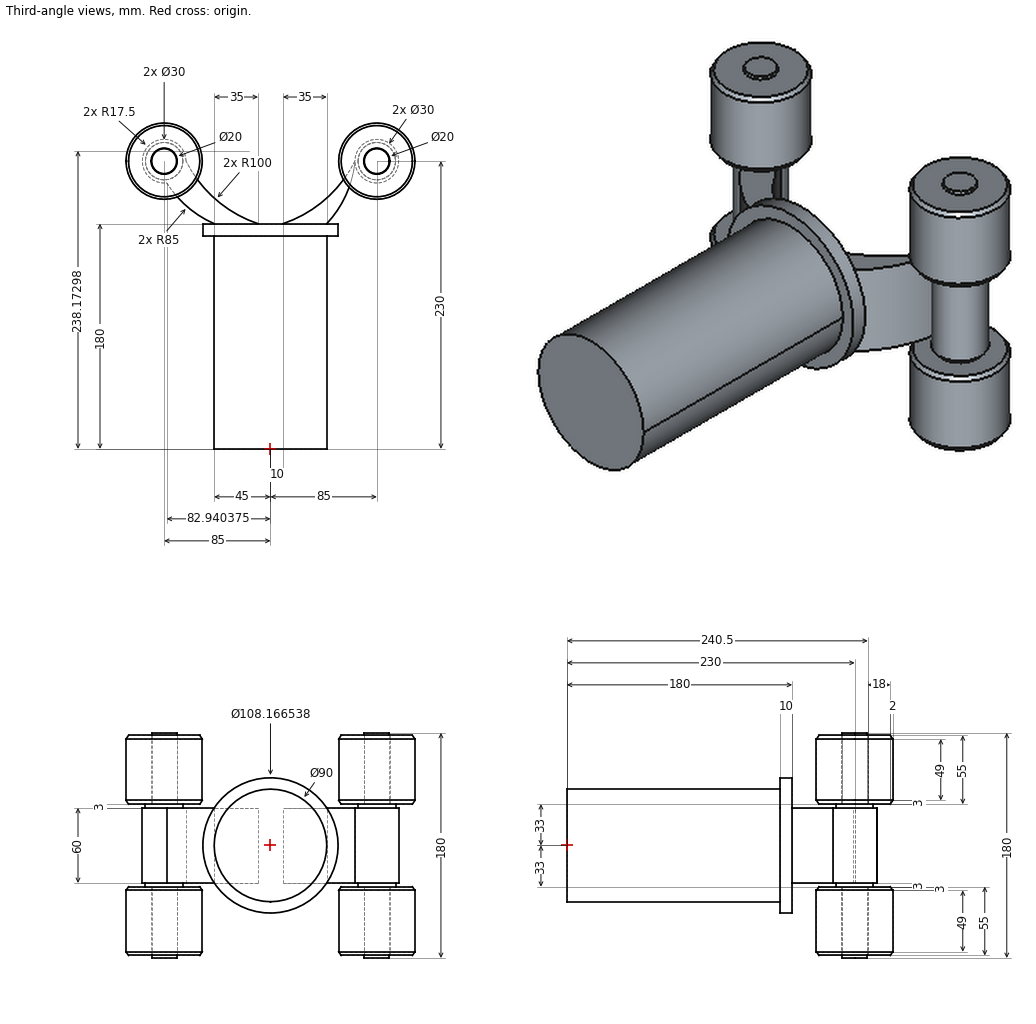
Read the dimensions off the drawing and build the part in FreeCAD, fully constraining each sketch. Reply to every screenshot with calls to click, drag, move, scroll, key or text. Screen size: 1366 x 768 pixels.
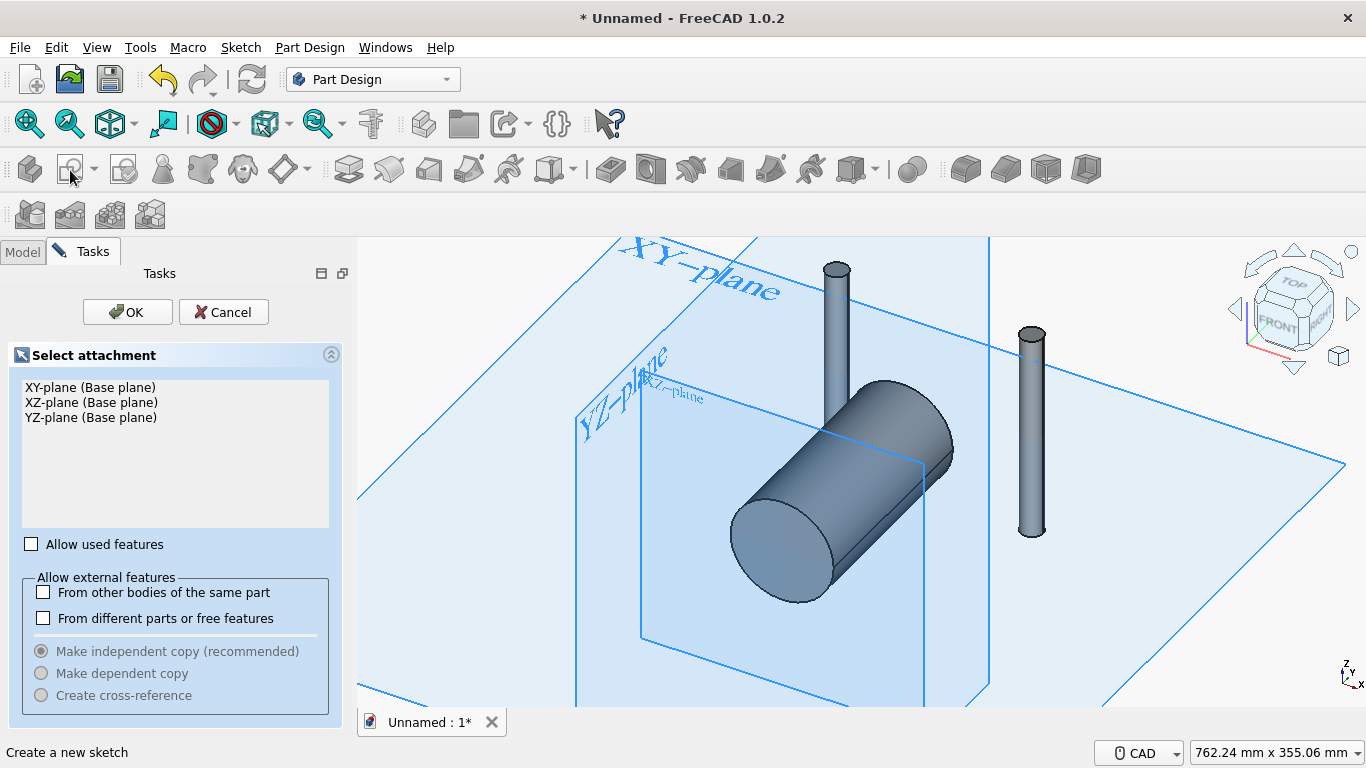
click(82, 388)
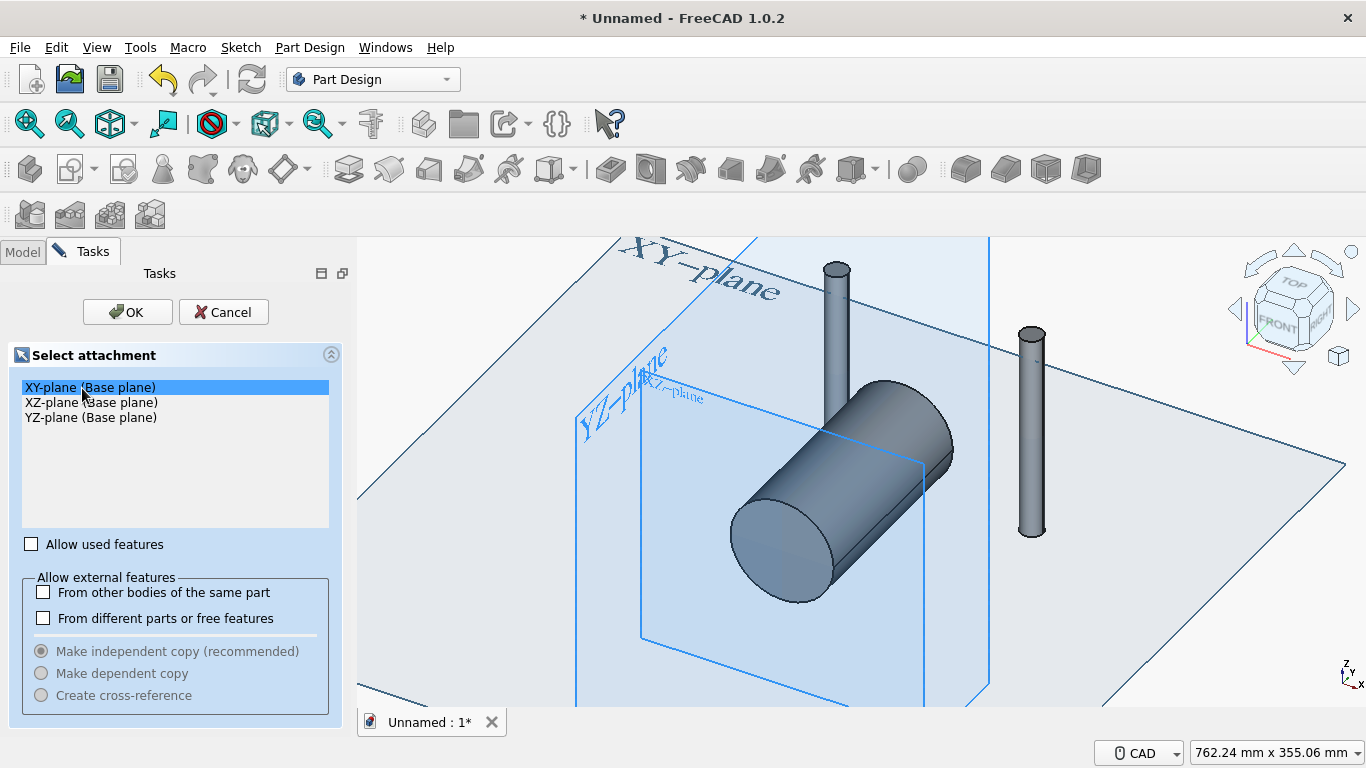
click(128, 312)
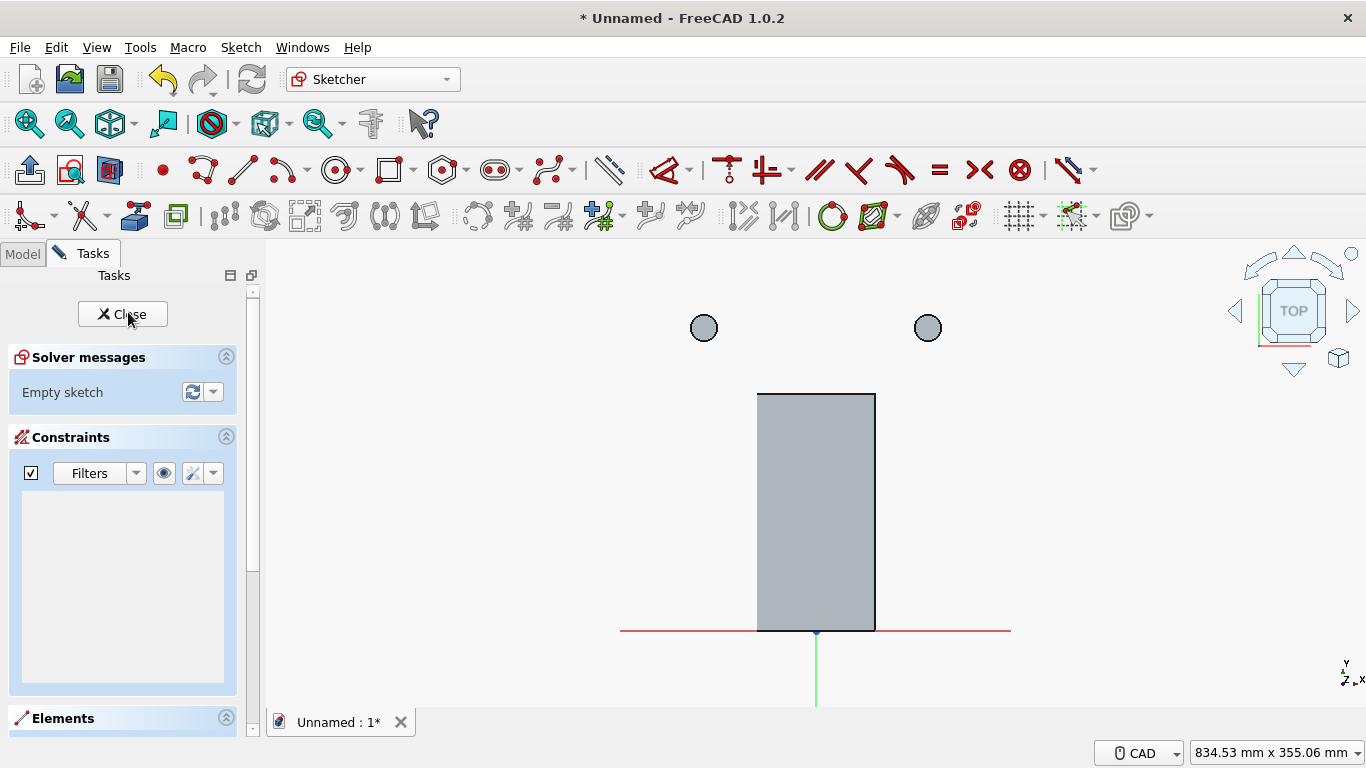
click(110, 170)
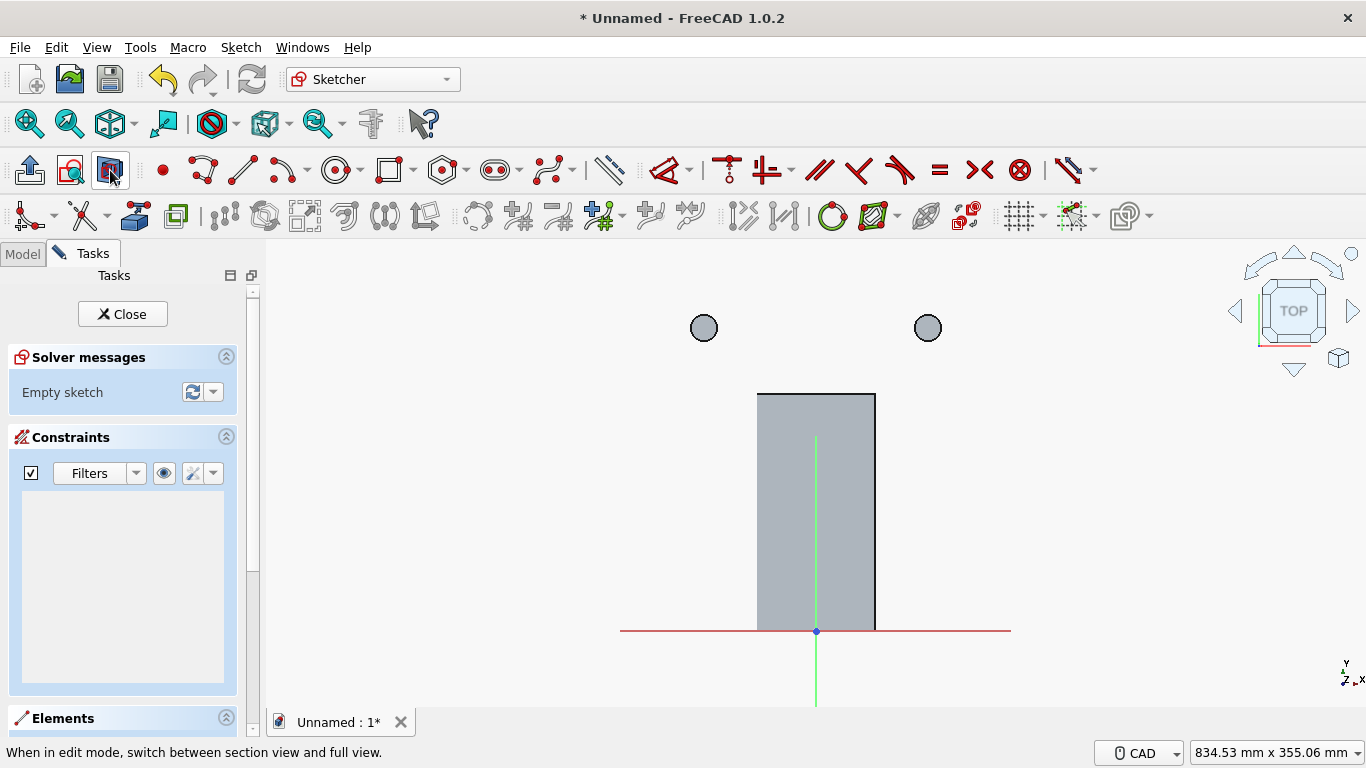
click(244, 170)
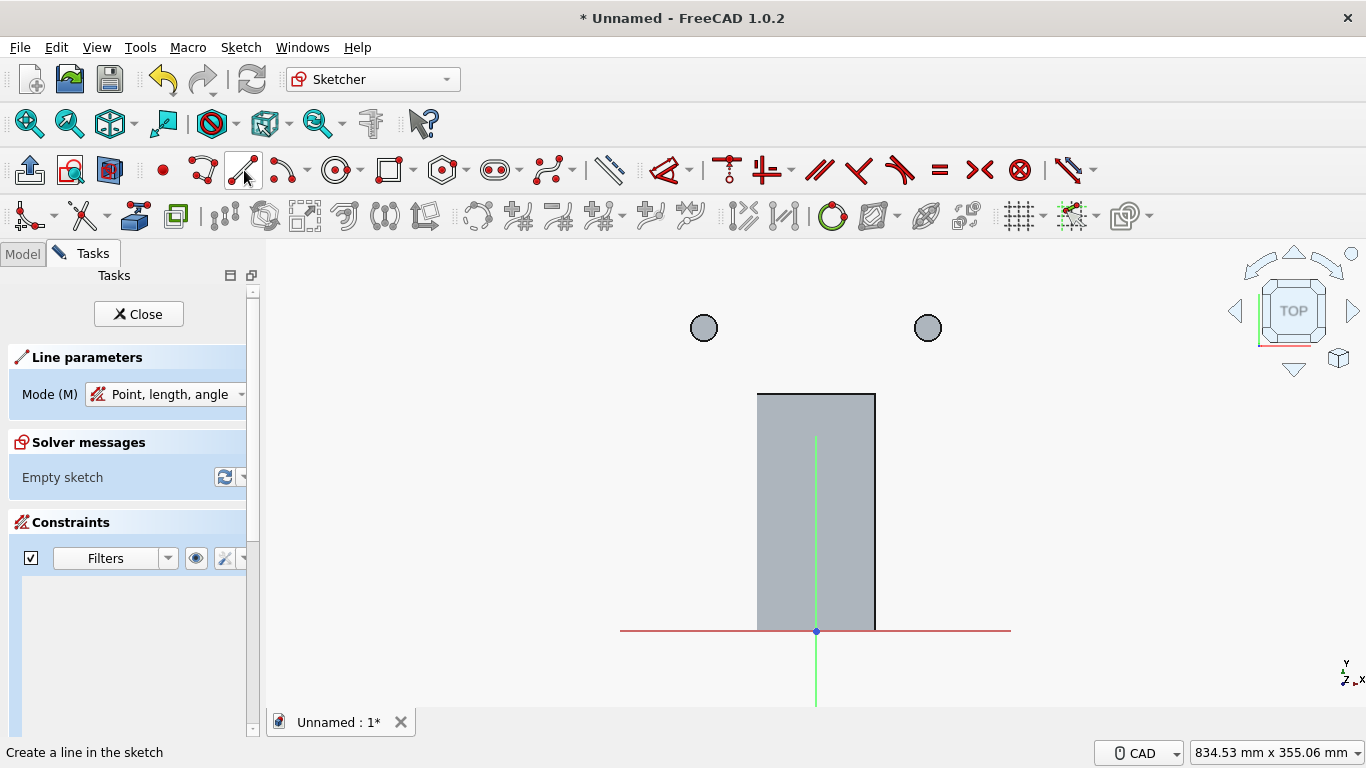
click(757, 394)
click(803, 394)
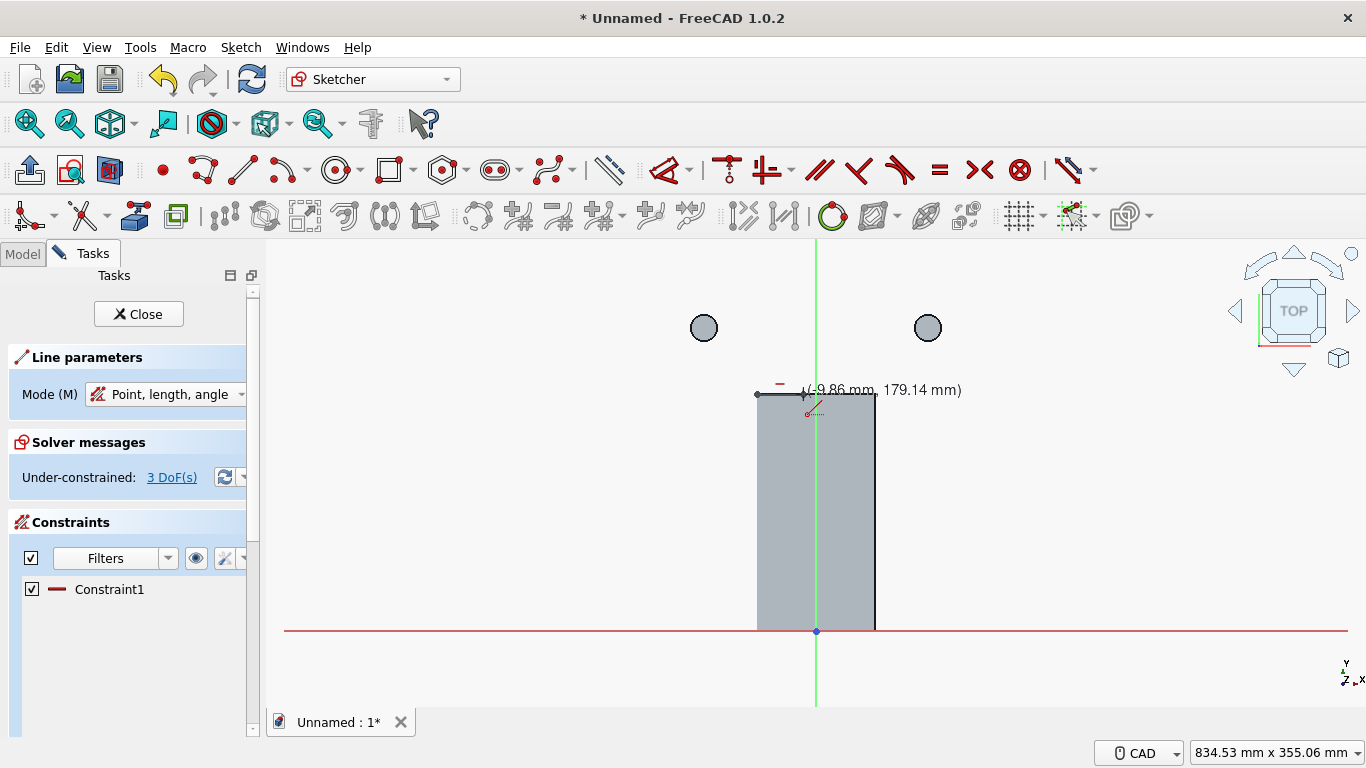
key(g)
key(3)
key(a)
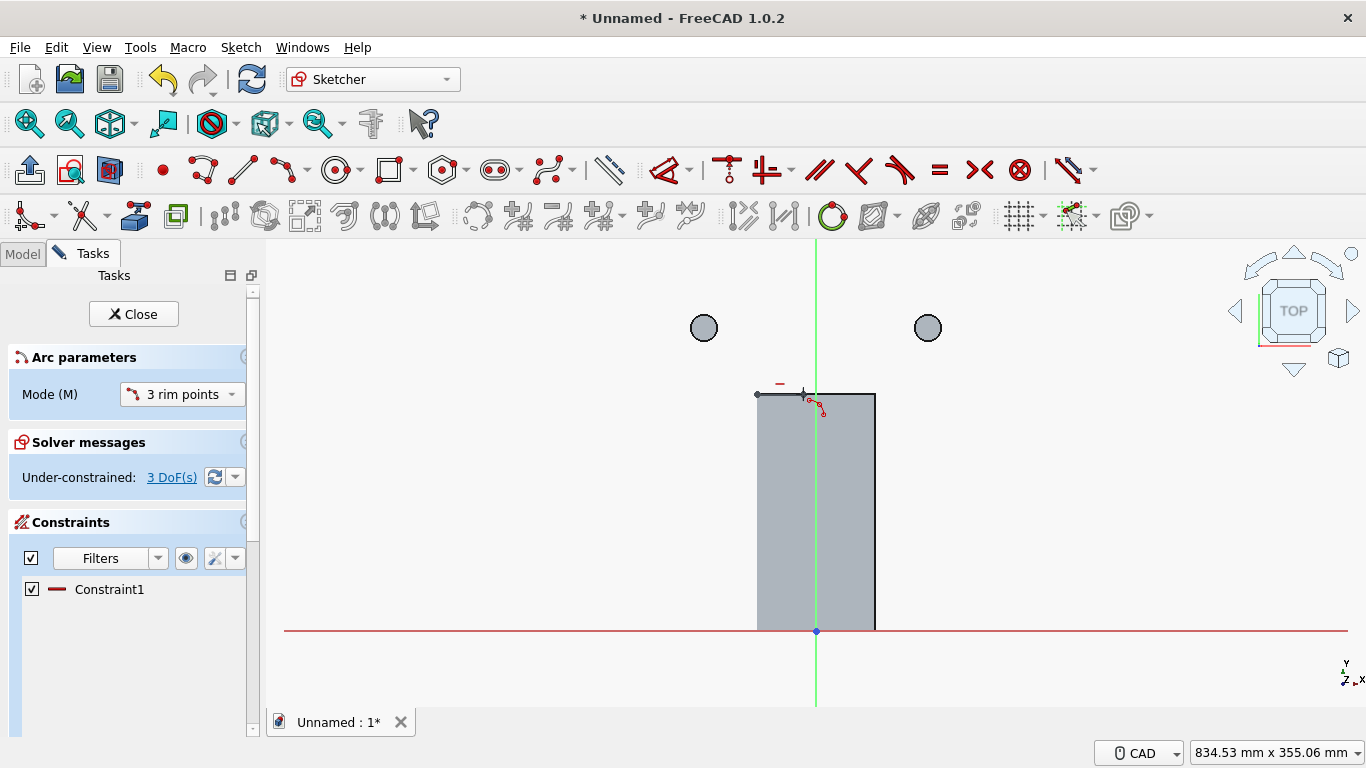
click(803, 395)
click(727, 328)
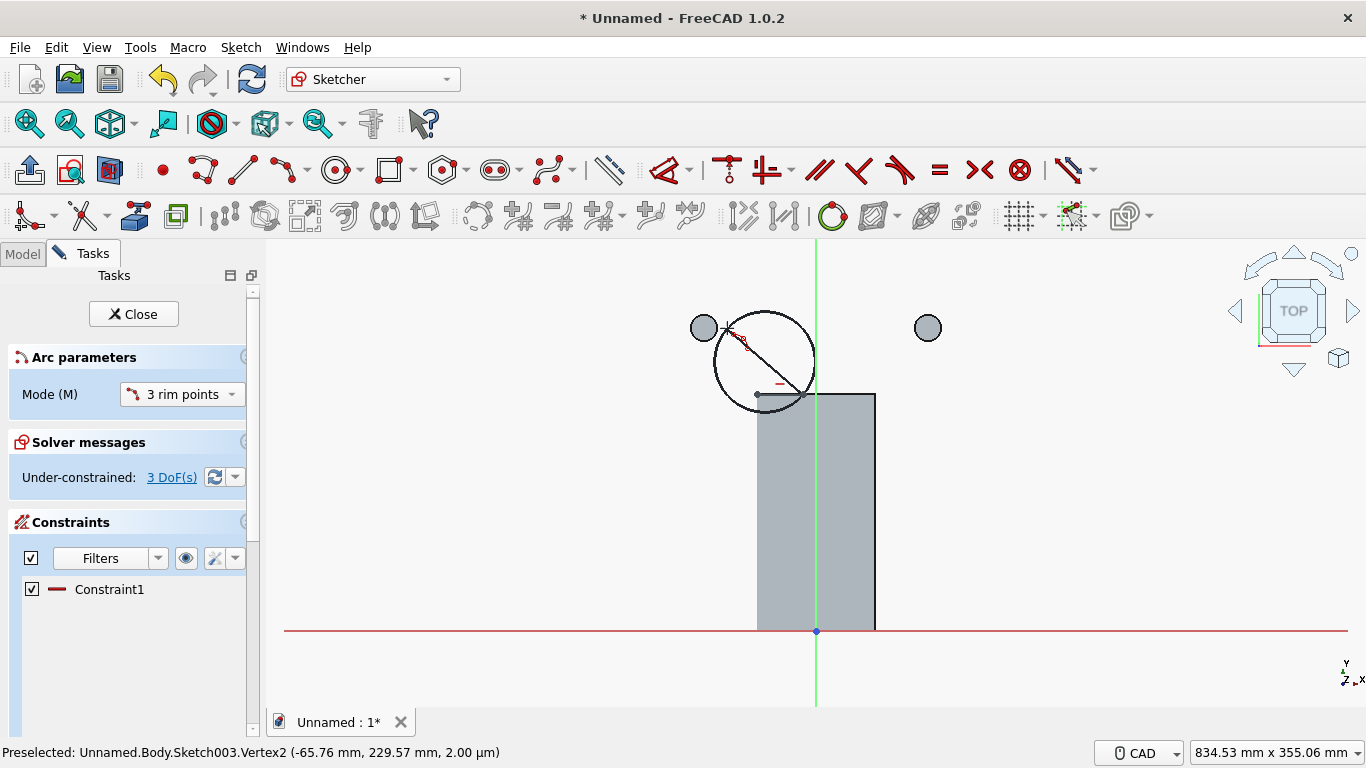
scroll(758, 368, up, 3)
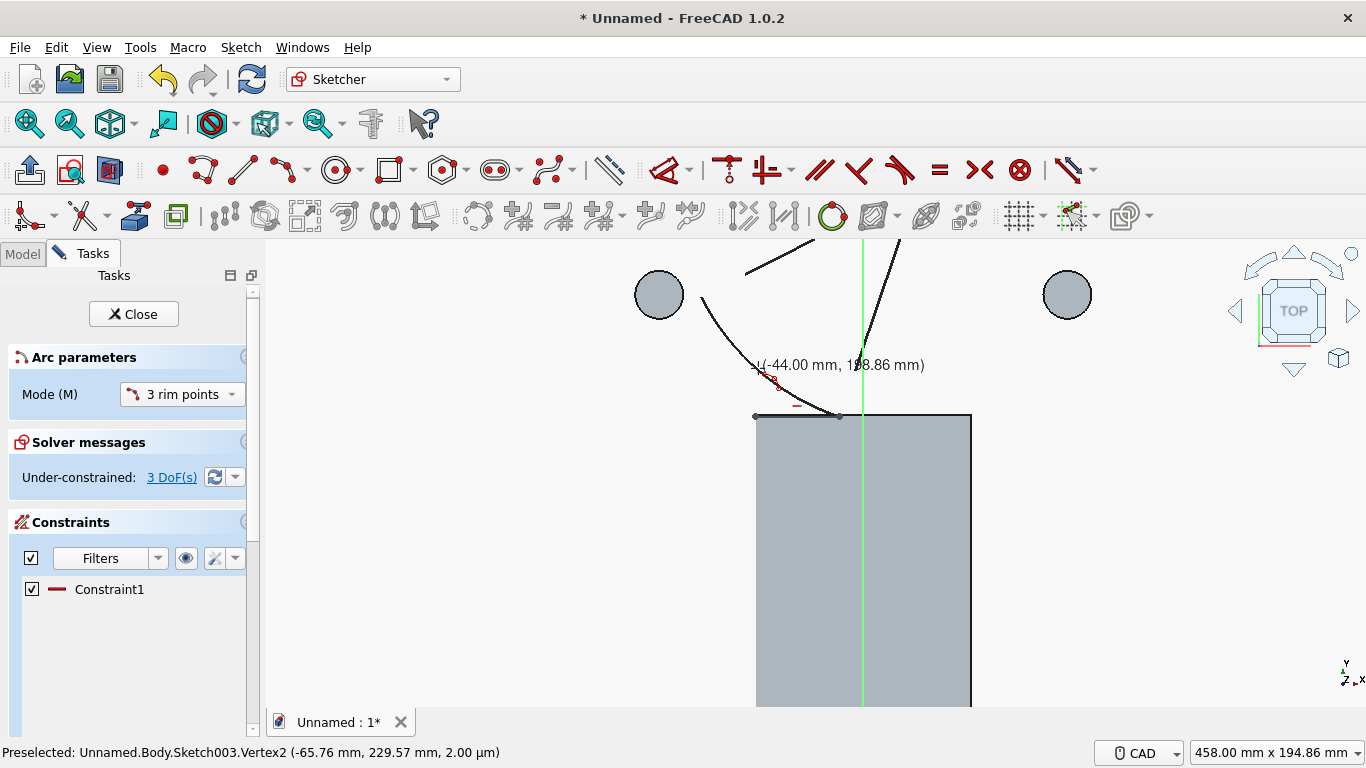
click(758, 369)